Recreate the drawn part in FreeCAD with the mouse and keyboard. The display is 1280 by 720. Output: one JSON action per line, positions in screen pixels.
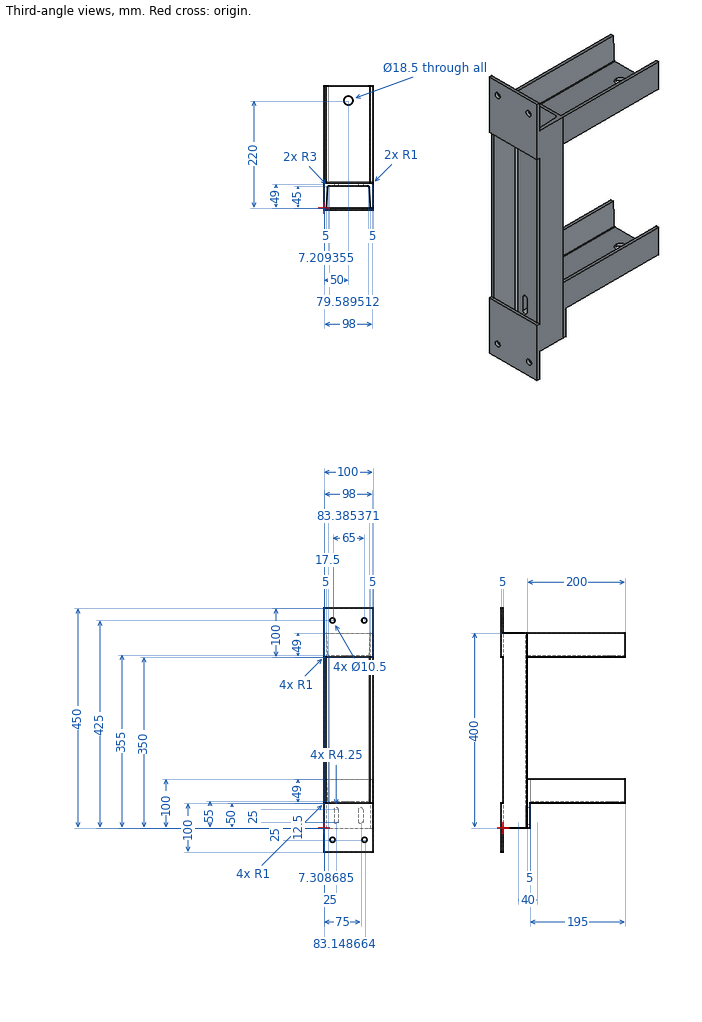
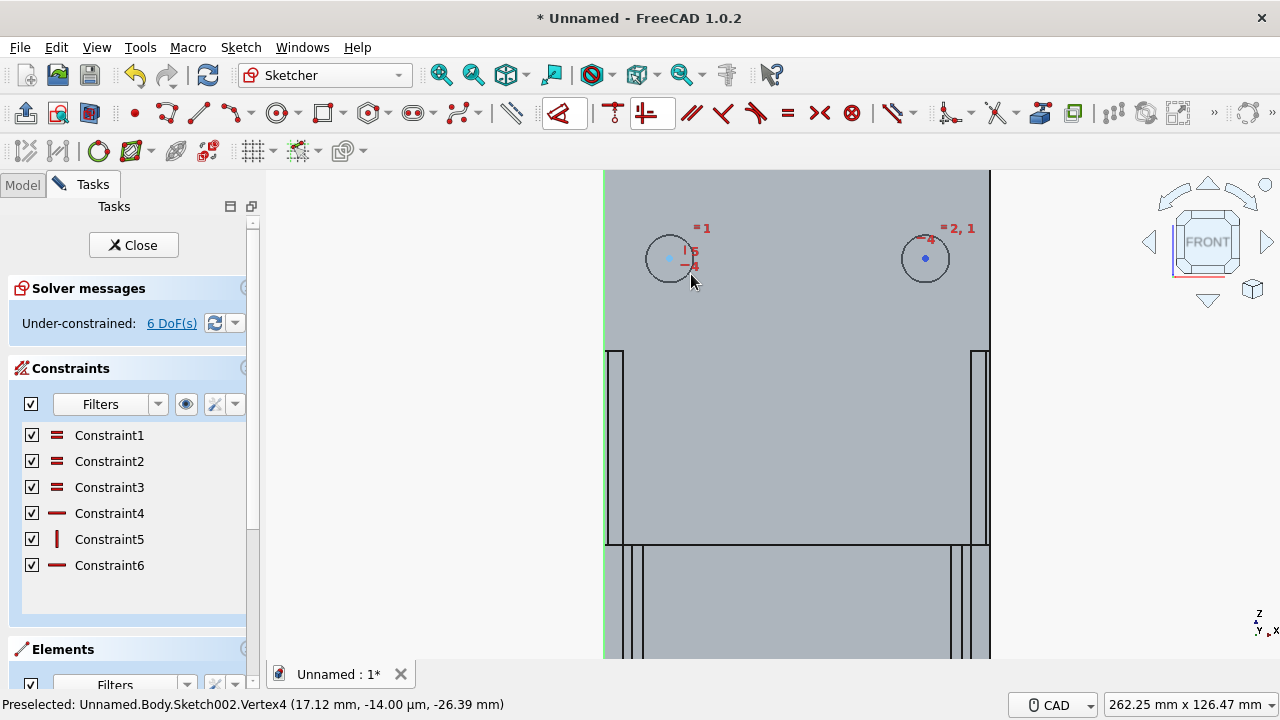
{"action": "left_click", "coordinate": [687, 276]}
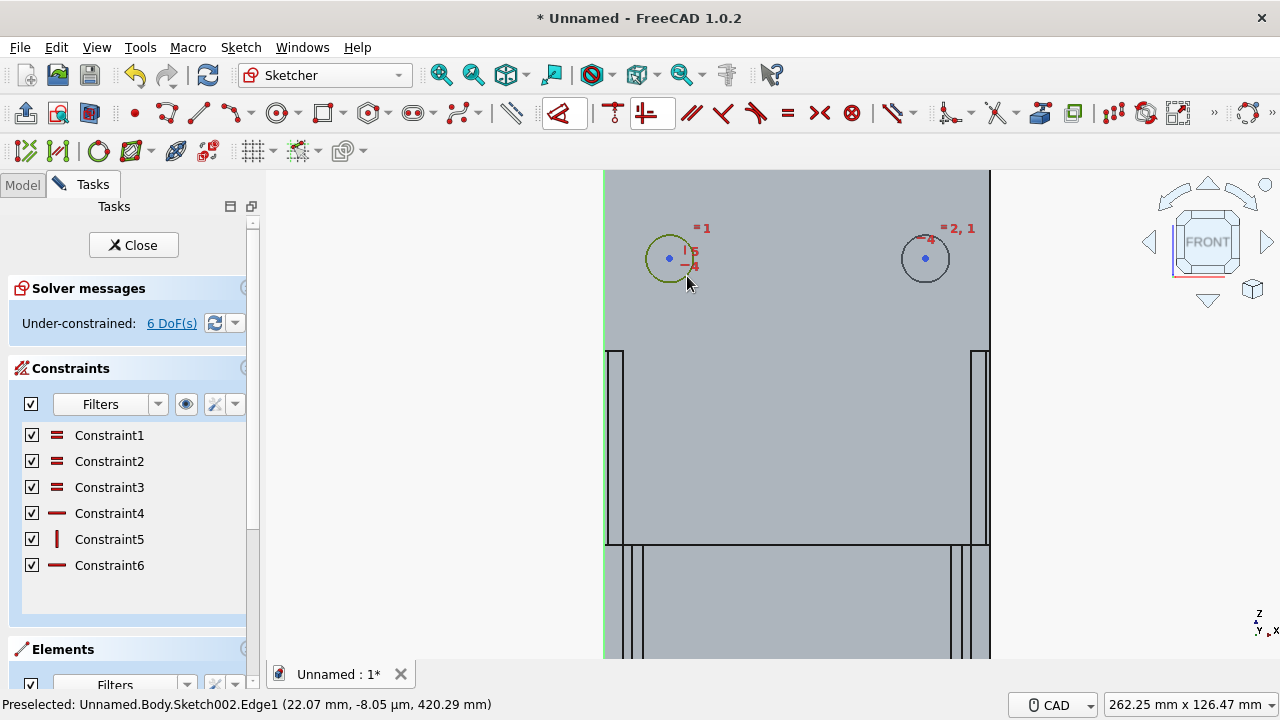
{"action": "key", "text": "k o"}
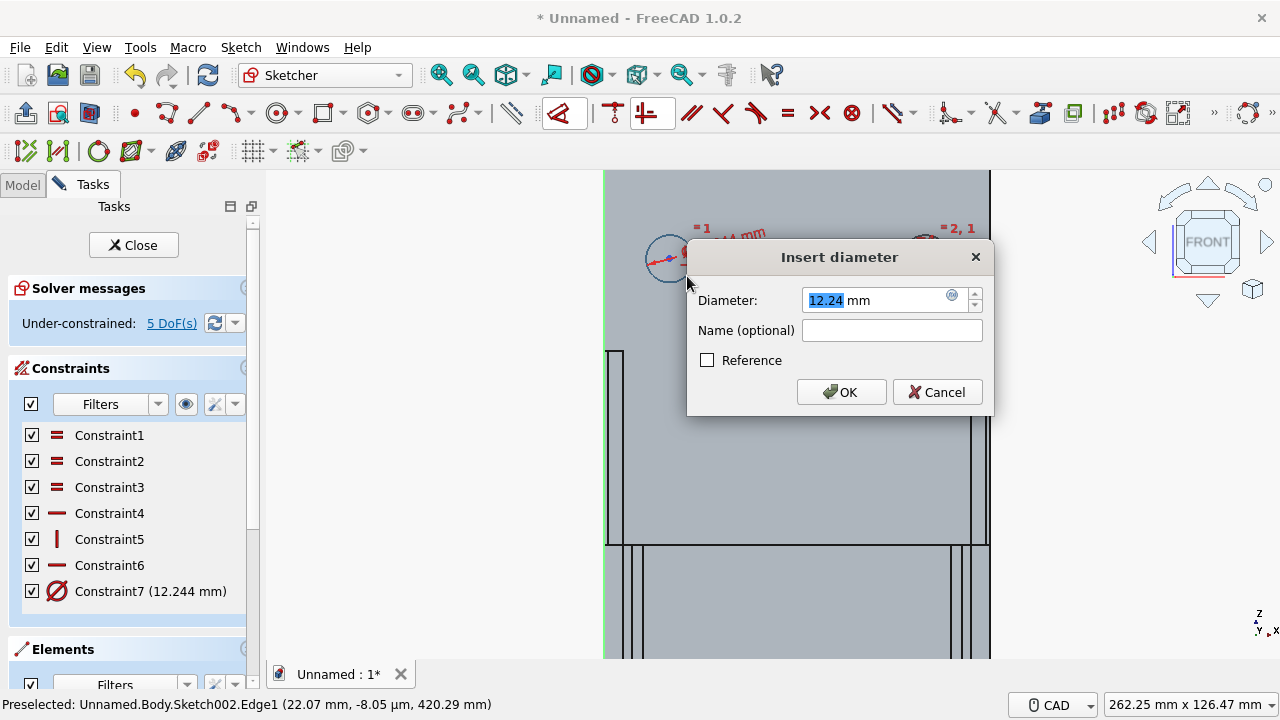
{"action": "type", "text": "10.5"}
{"action": "key", "text": "Return"}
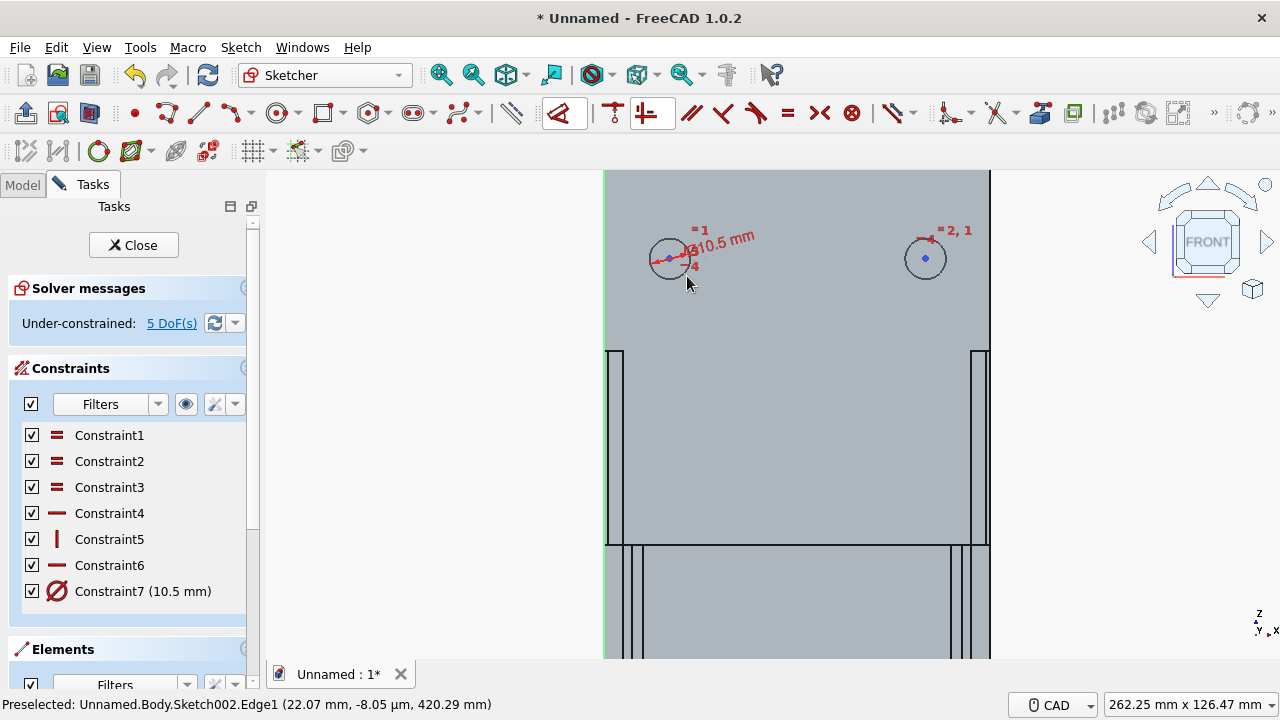
{"action": "scroll", "coordinate": [691, 274], "scroll_direction": "down", "scroll_amount": 9}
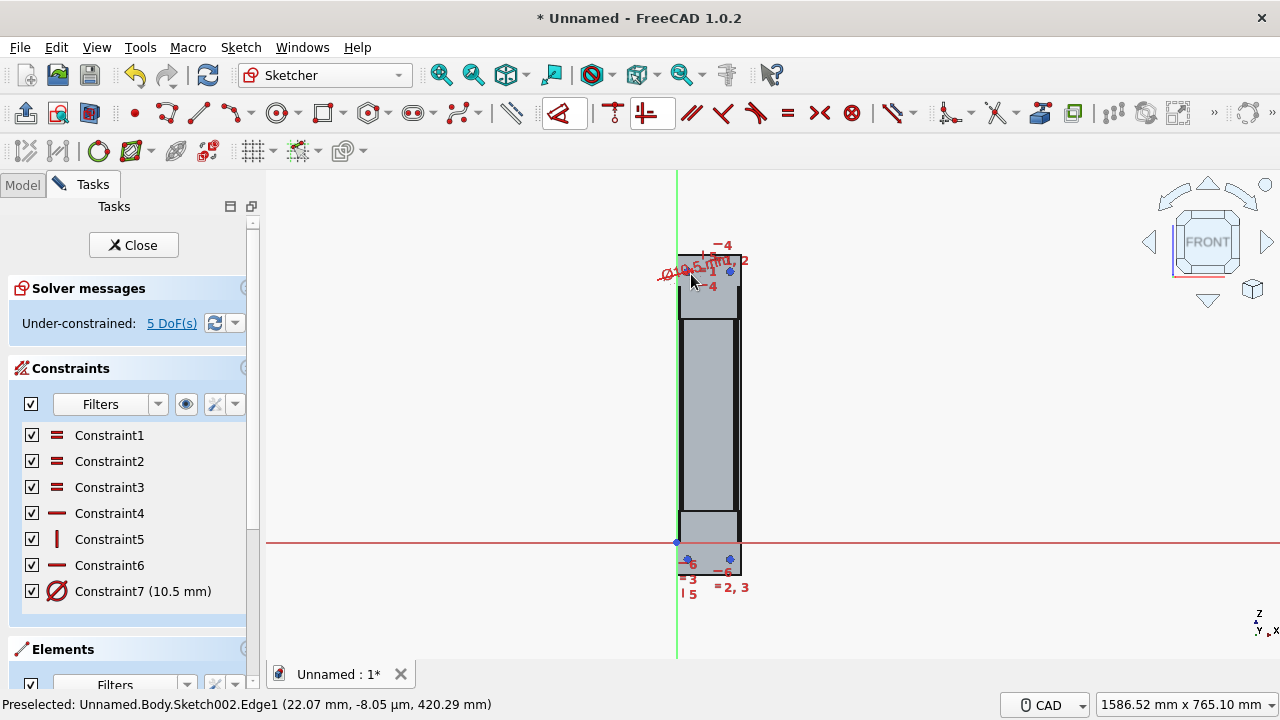
{"action": "scroll", "coordinate": [730, 560], "scroll_direction": "up", "scroll_amount": 5}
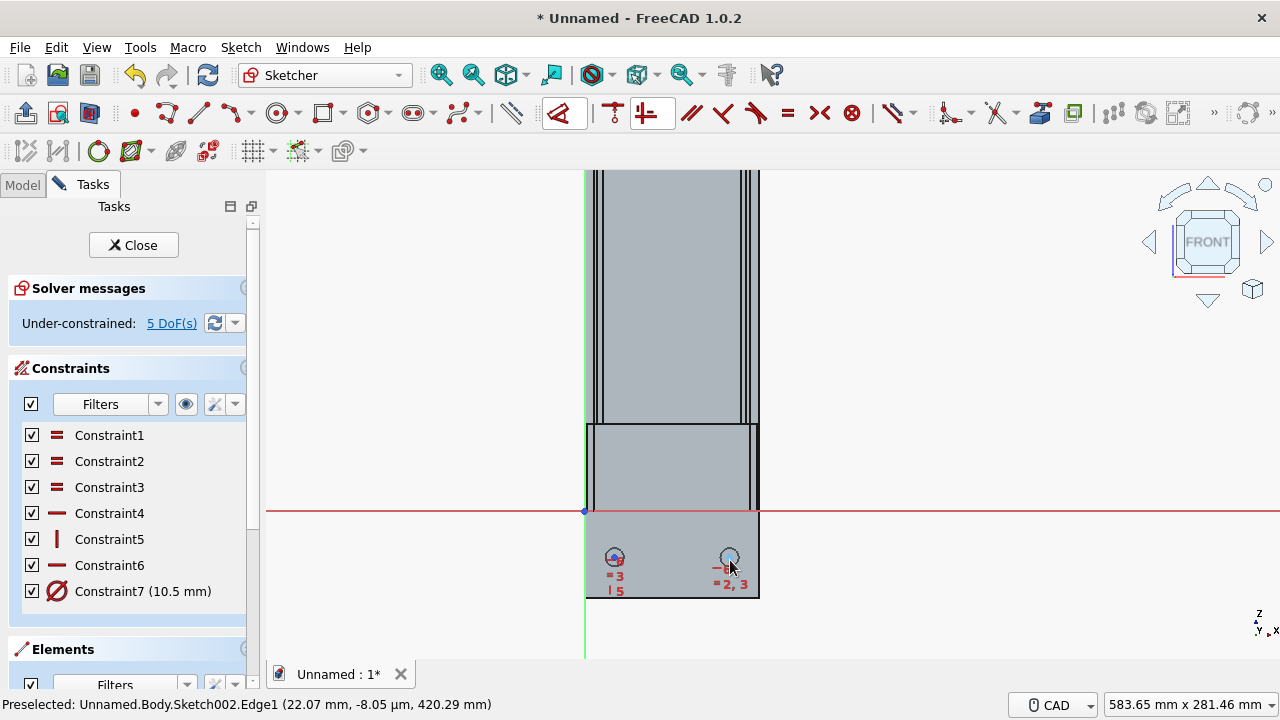
{"action": "left_click", "coordinate": [730, 557]}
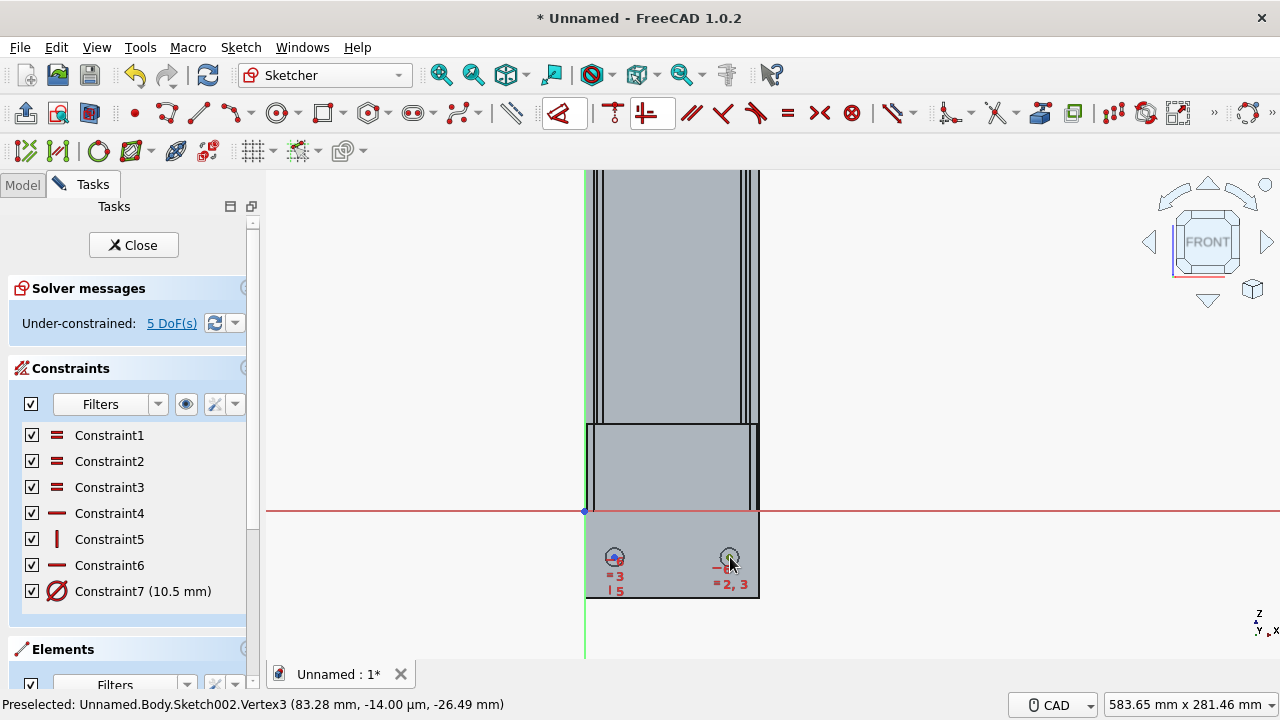
{"action": "key", "text": "i"}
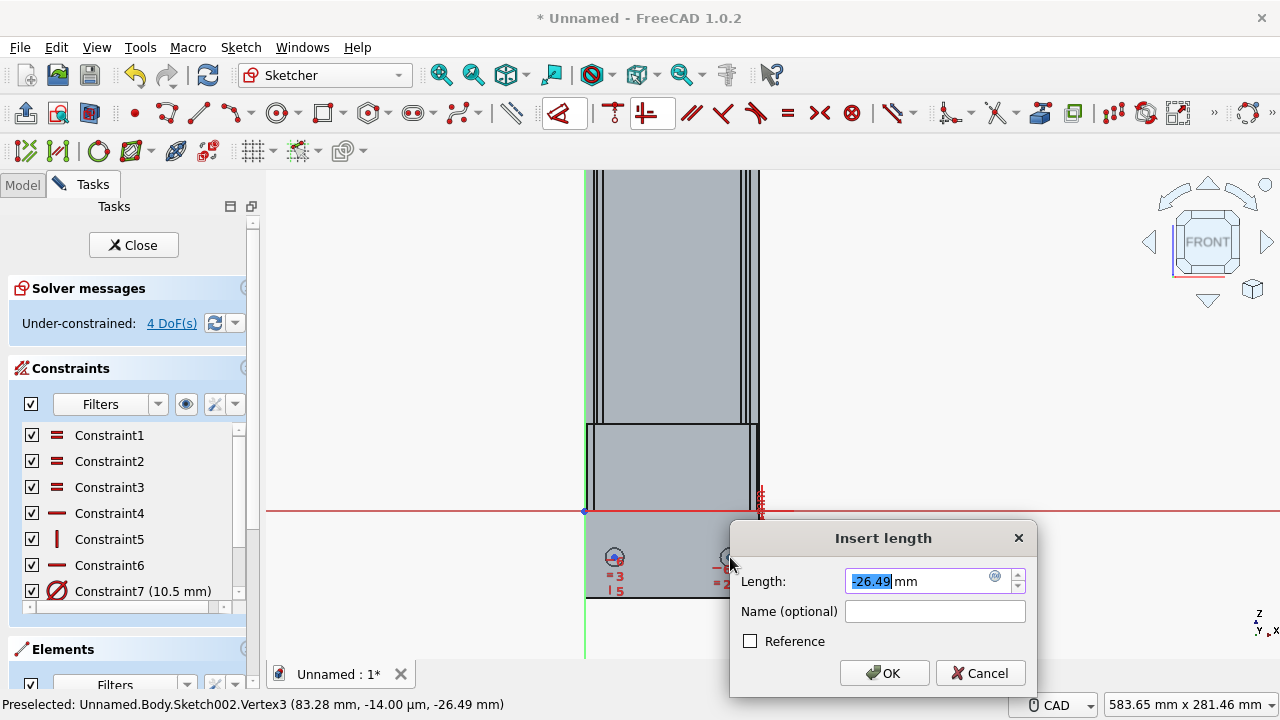
{"action": "type", "text": "-25"}
{"action": "key", "text": "Return"}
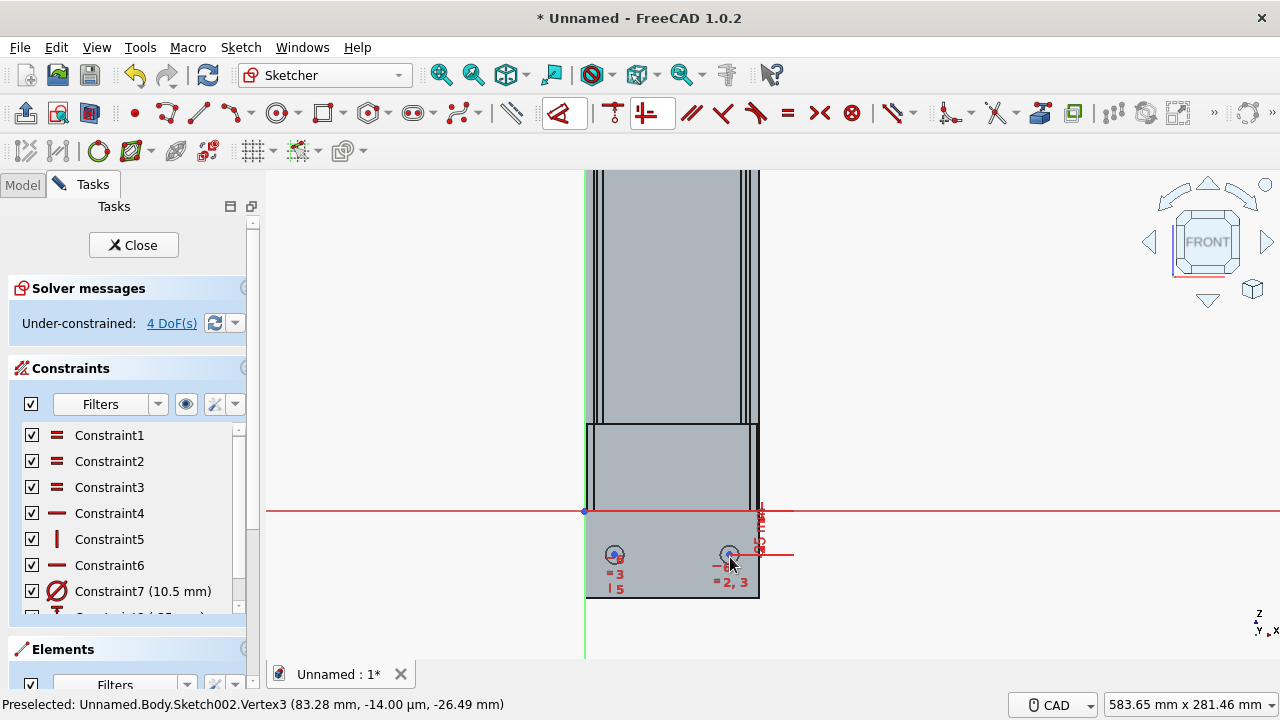
{"action": "scroll", "coordinate": [729, 560], "scroll_direction": "down", "scroll_amount": 5}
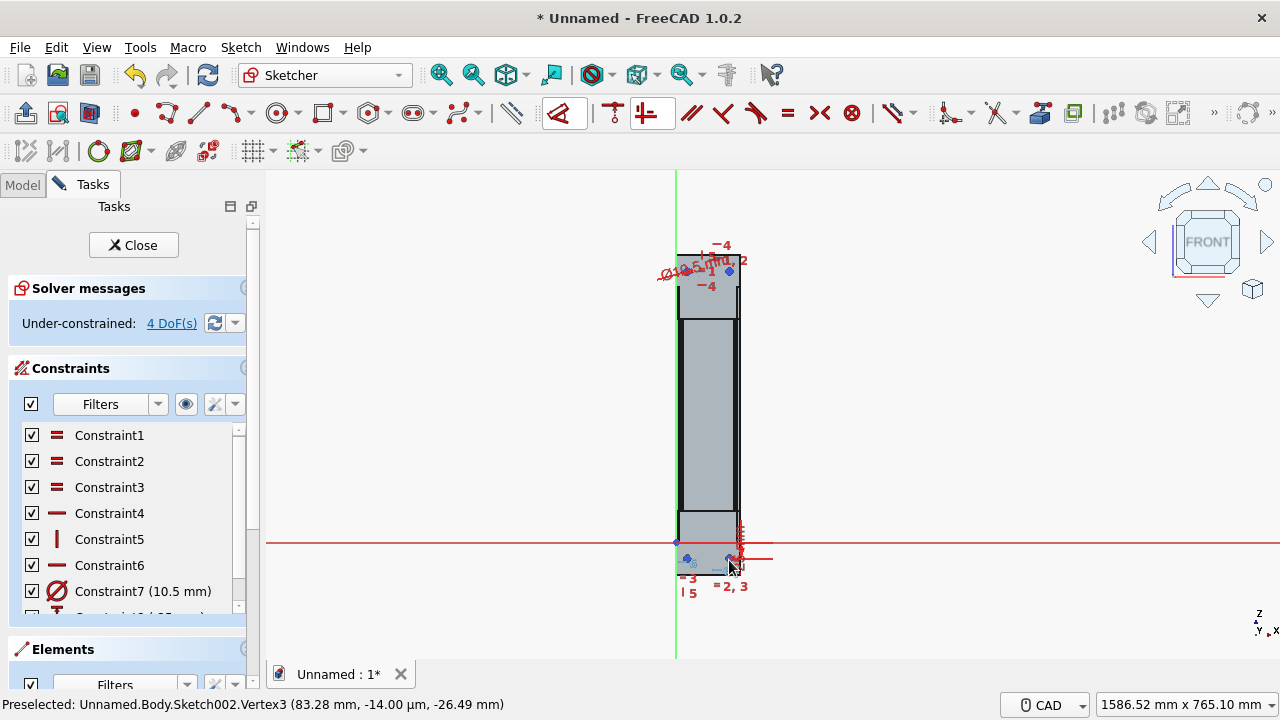
{"action": "left_click", "coordinate": [687, 272]}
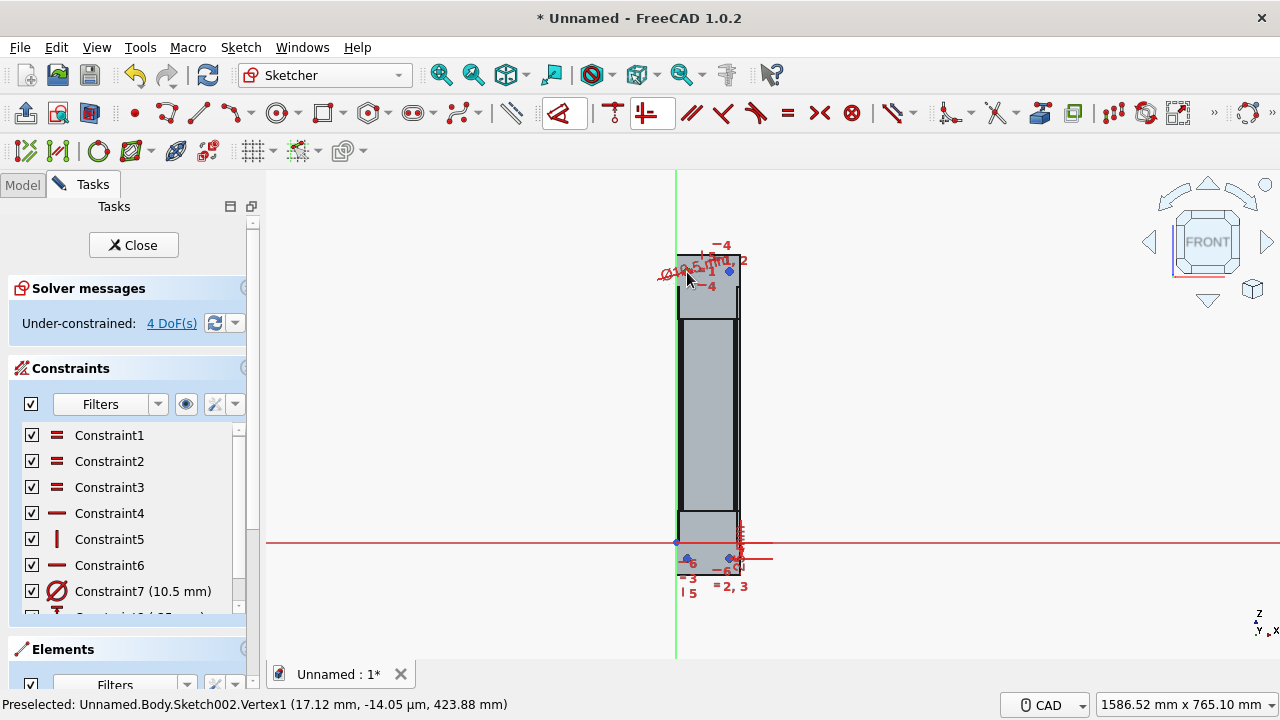
{"action": "key", "text": "i"}